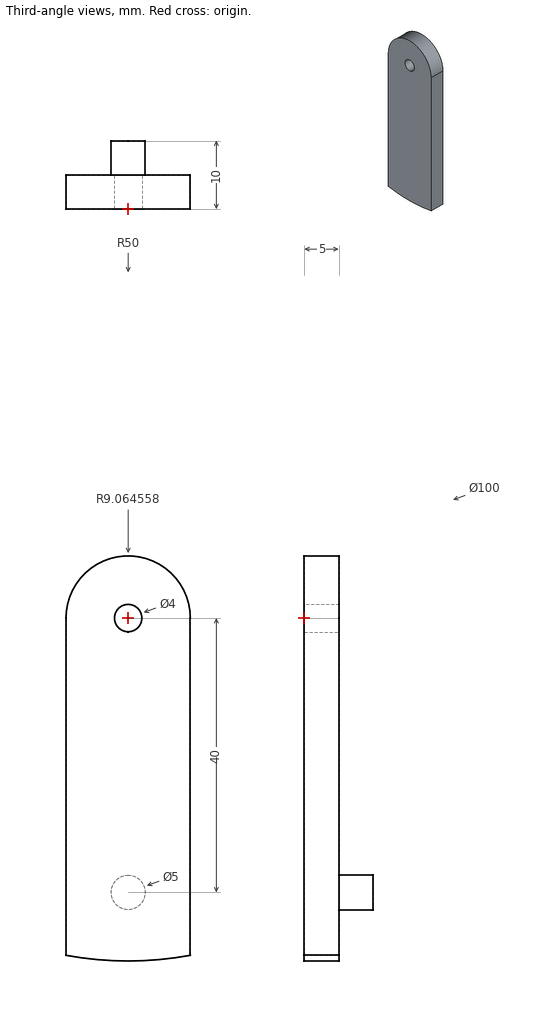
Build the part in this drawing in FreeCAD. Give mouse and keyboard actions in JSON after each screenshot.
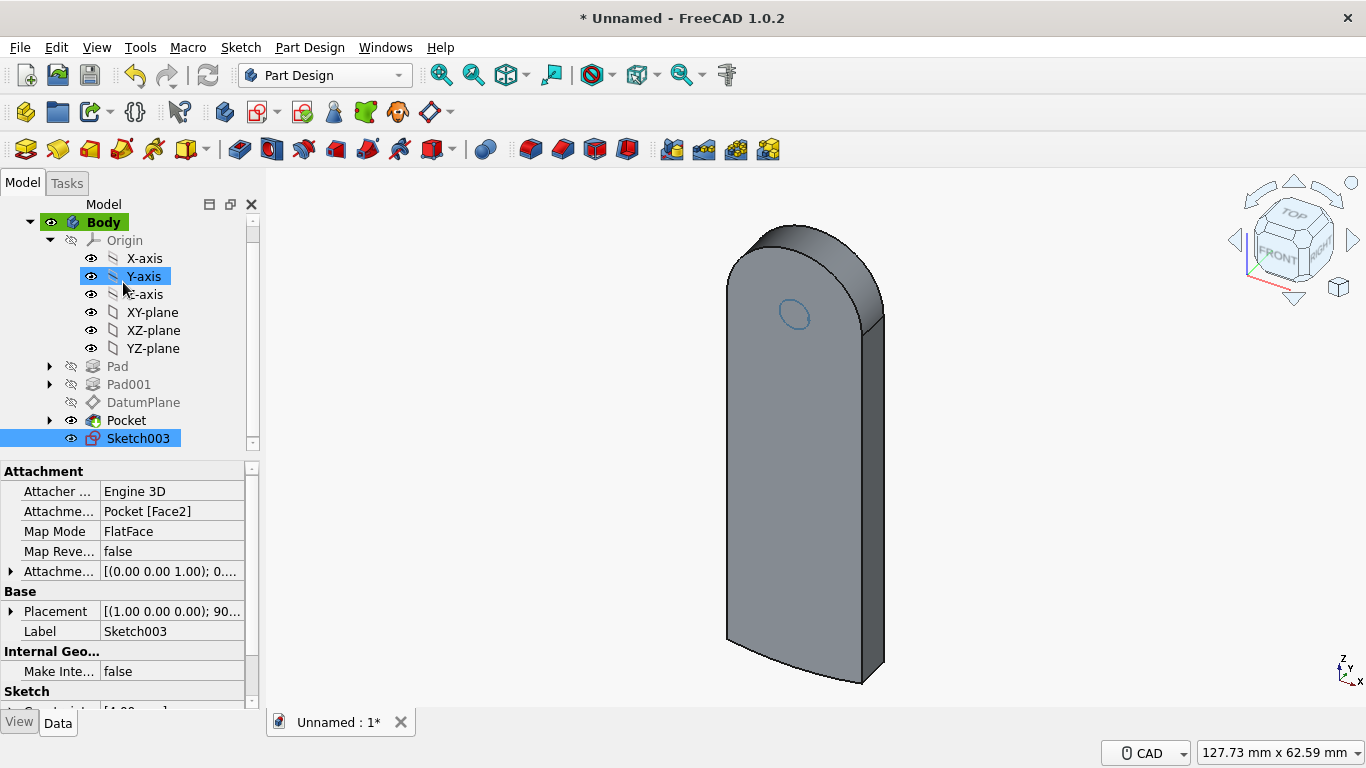
{"action": "left_click", "coordinate": [240, 150]}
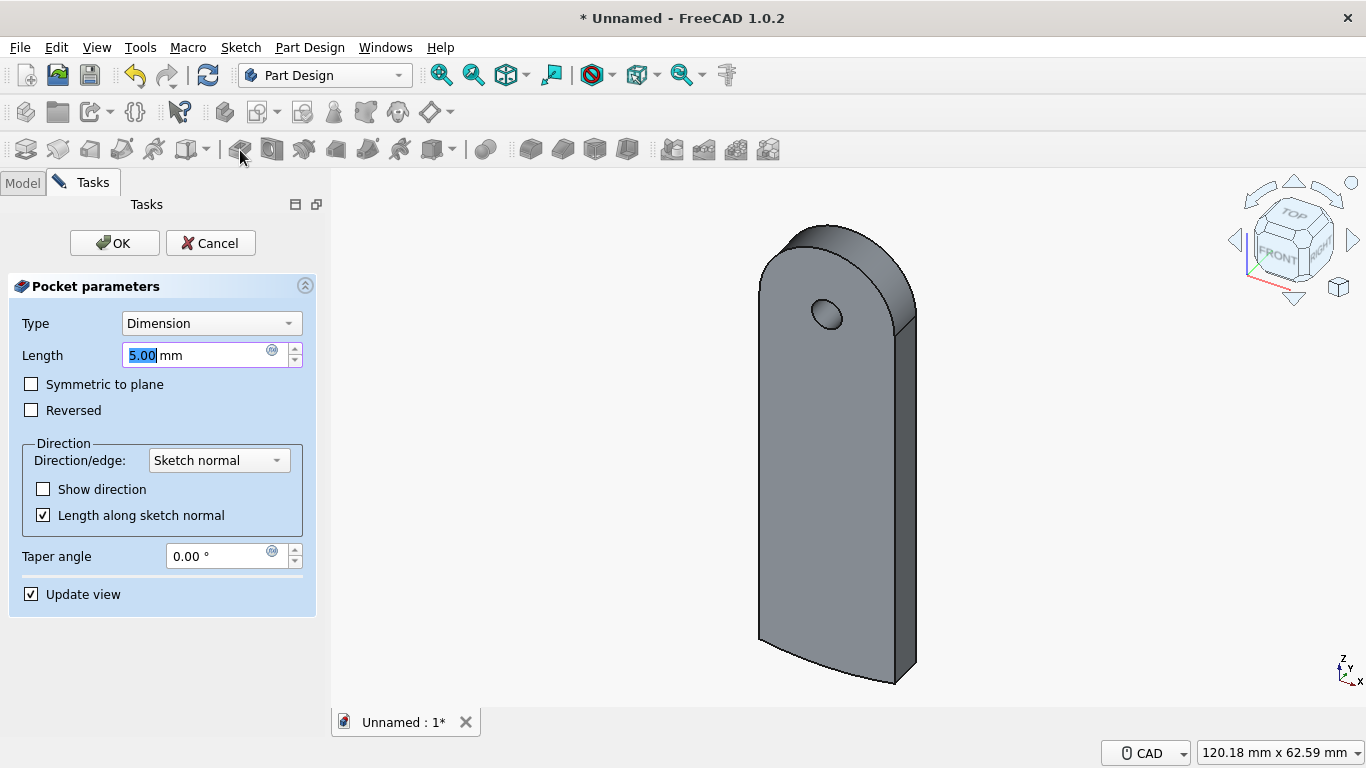
{"action": "left_click", "coordinate": [212, 324]}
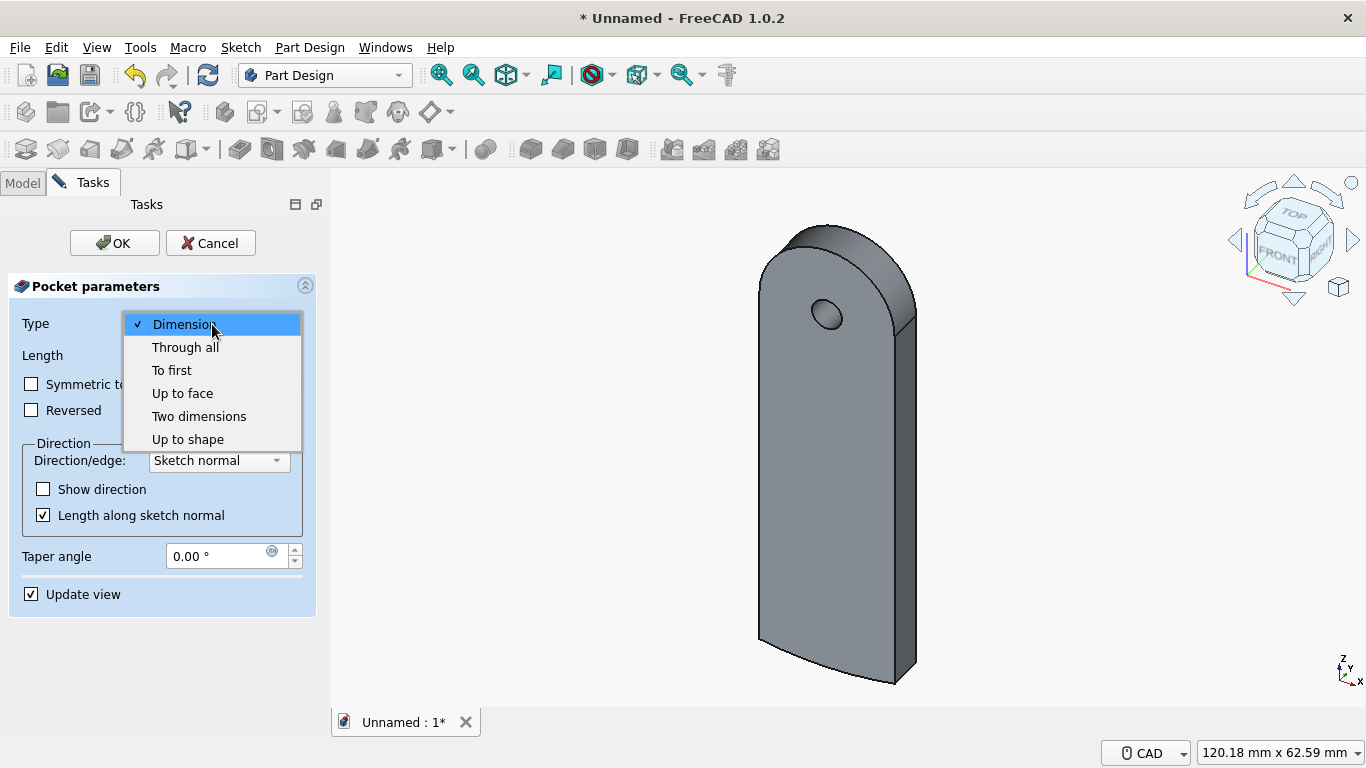
{"action": "left_click", "coordinate": [212, 348]}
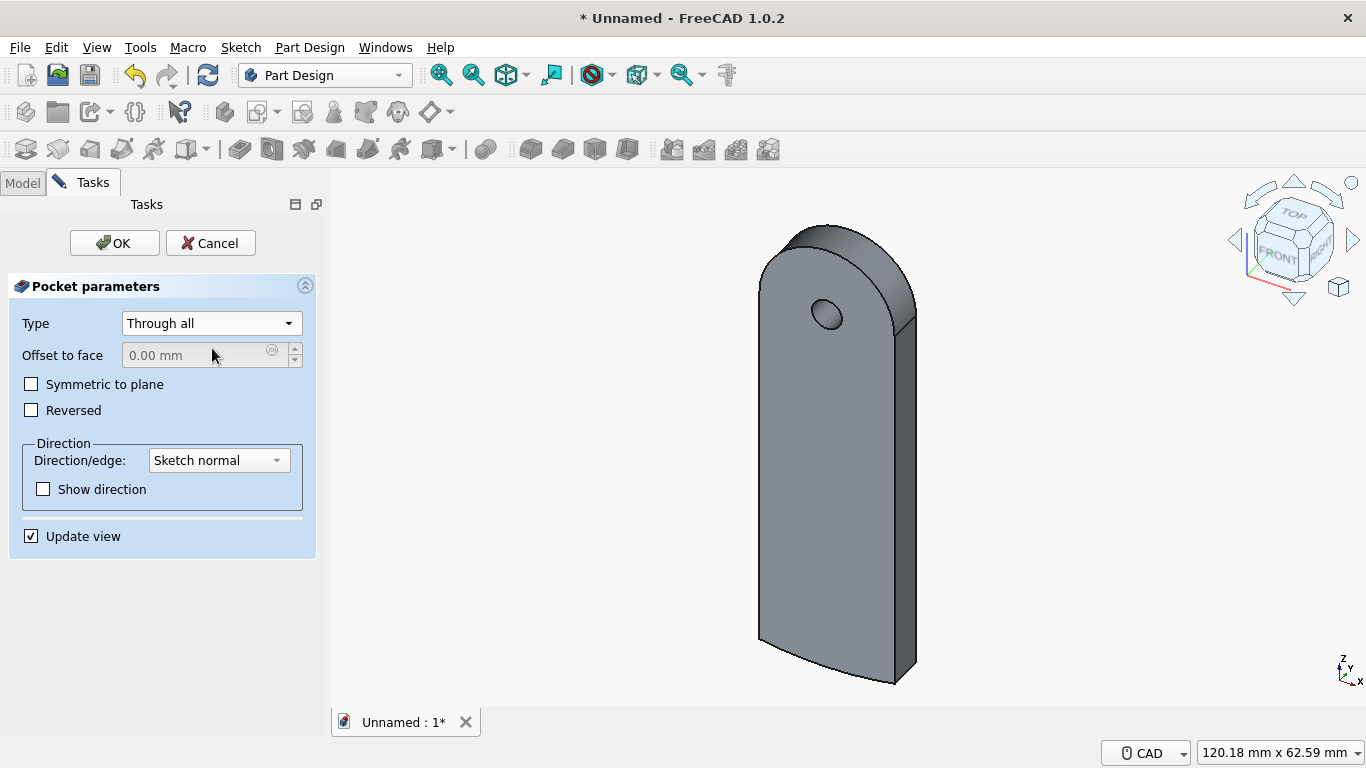
{"action": "left_click", "coordinate": [115, 243]}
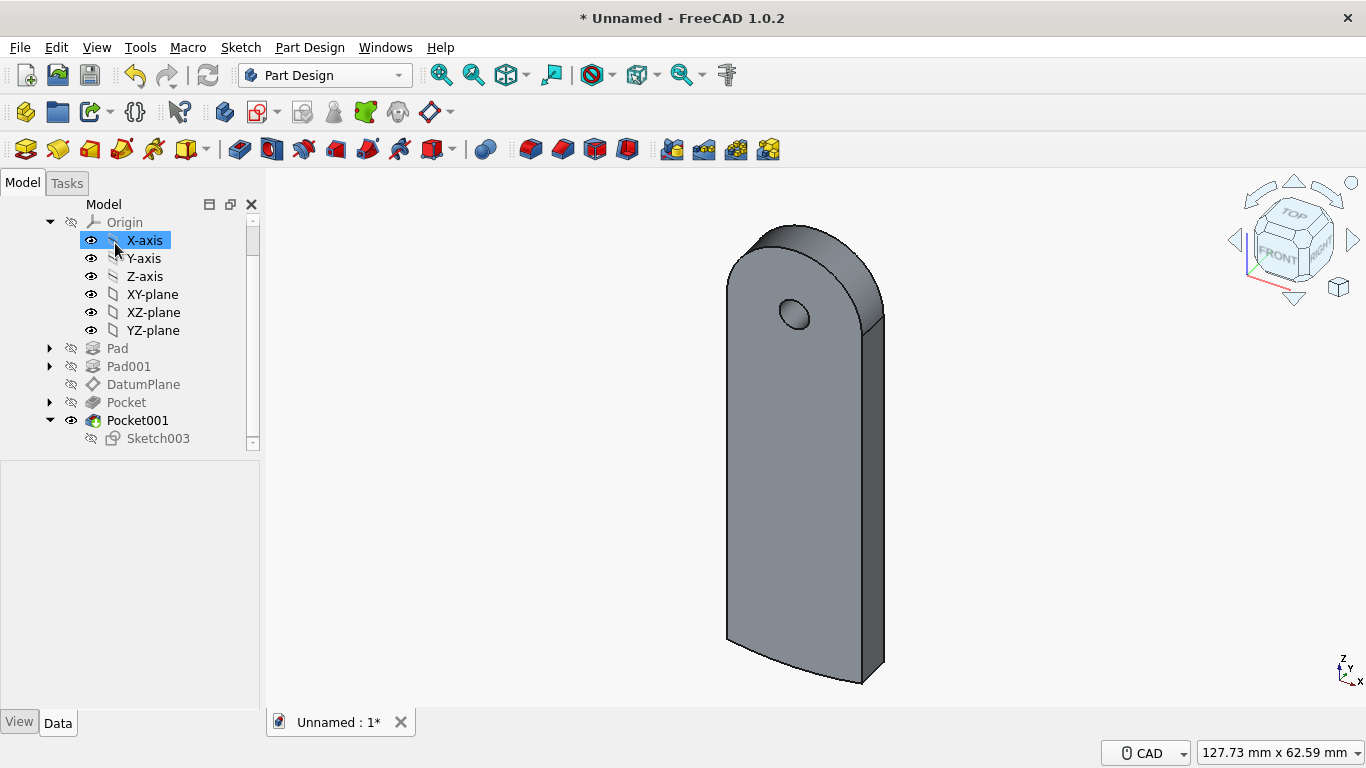
{"action": "key", "text": "0"}